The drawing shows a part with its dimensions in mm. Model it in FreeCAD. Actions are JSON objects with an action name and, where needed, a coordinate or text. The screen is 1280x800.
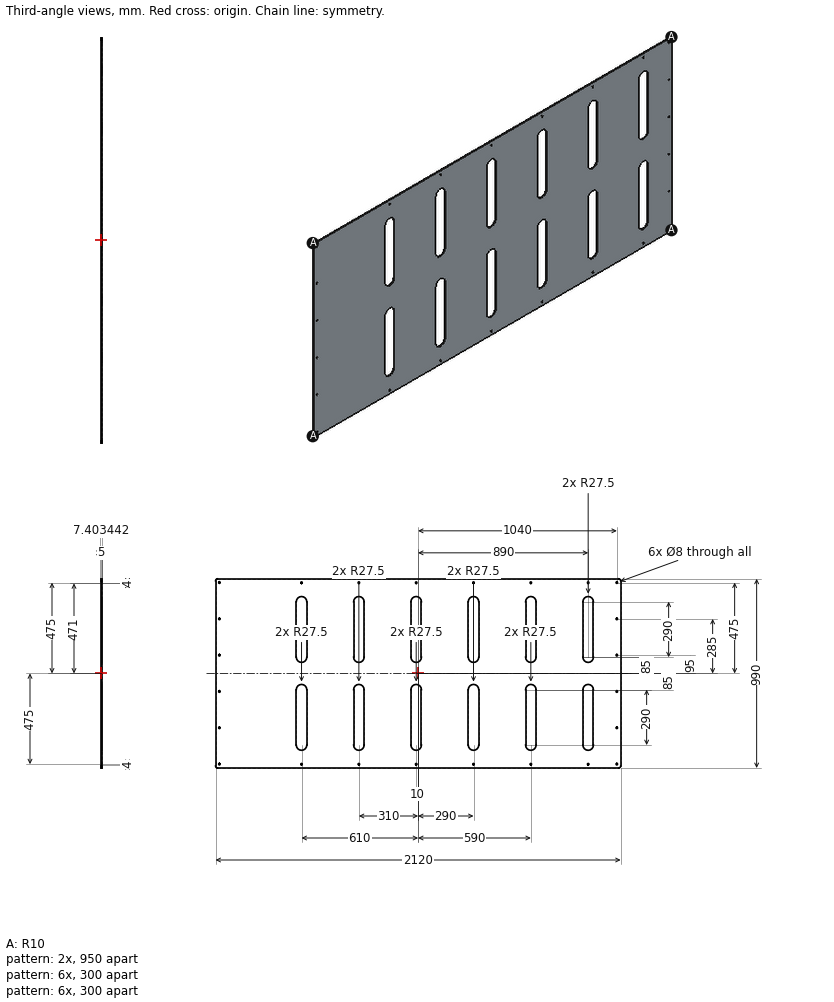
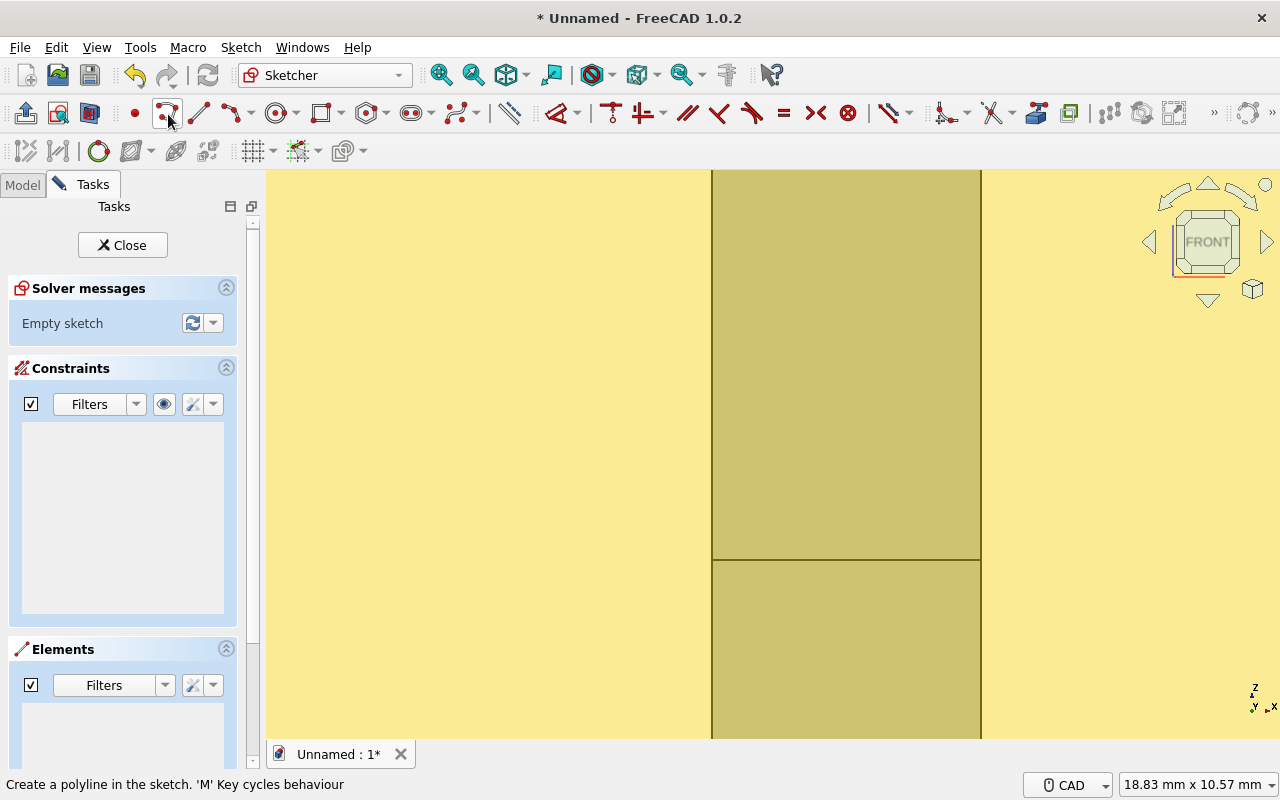
{"action": "left_click", "coordinate": [582, 345]}
{"action": "left_click", "coordinate": [981, 345]}
{"action": "left_click", "coordinate": [981, 560]}
{"action": "left_click", "coordinate": [712, 560]}
{"action": "left_click", "coordinate": [582, 346]}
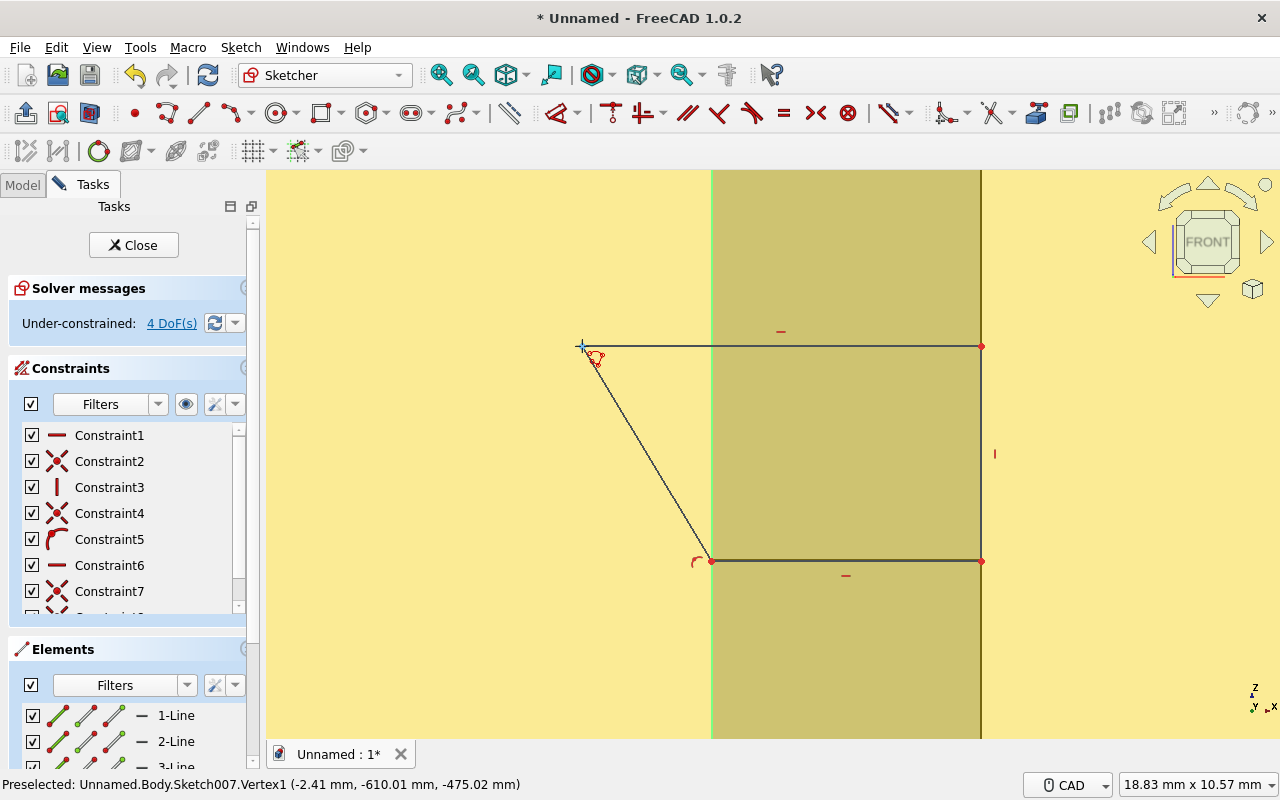
{"action": "left_click", "coordinate": [200, 114]}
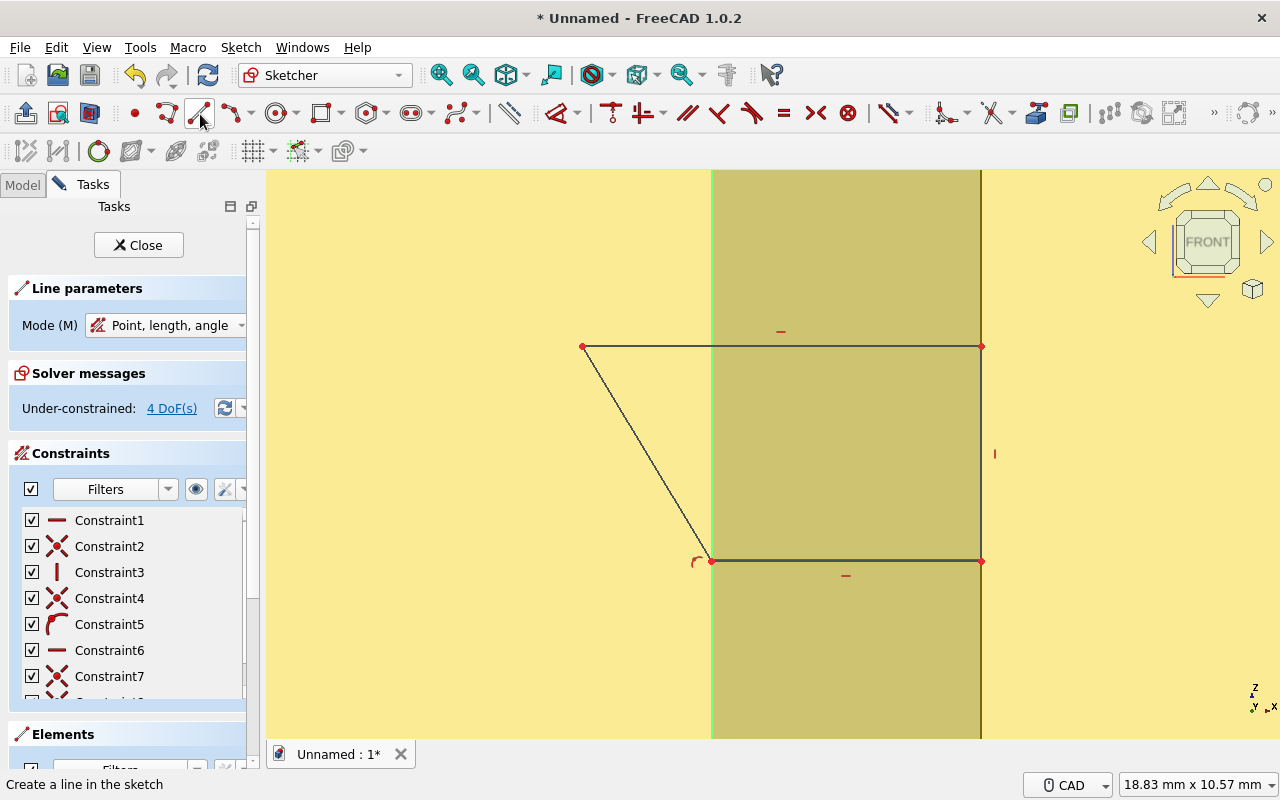
{"action": "left_click", "coordinate": [542, 345]}
{"action": "left_click", "coordinate": [423, 345]}
{"action": "key", "text": "Escape"}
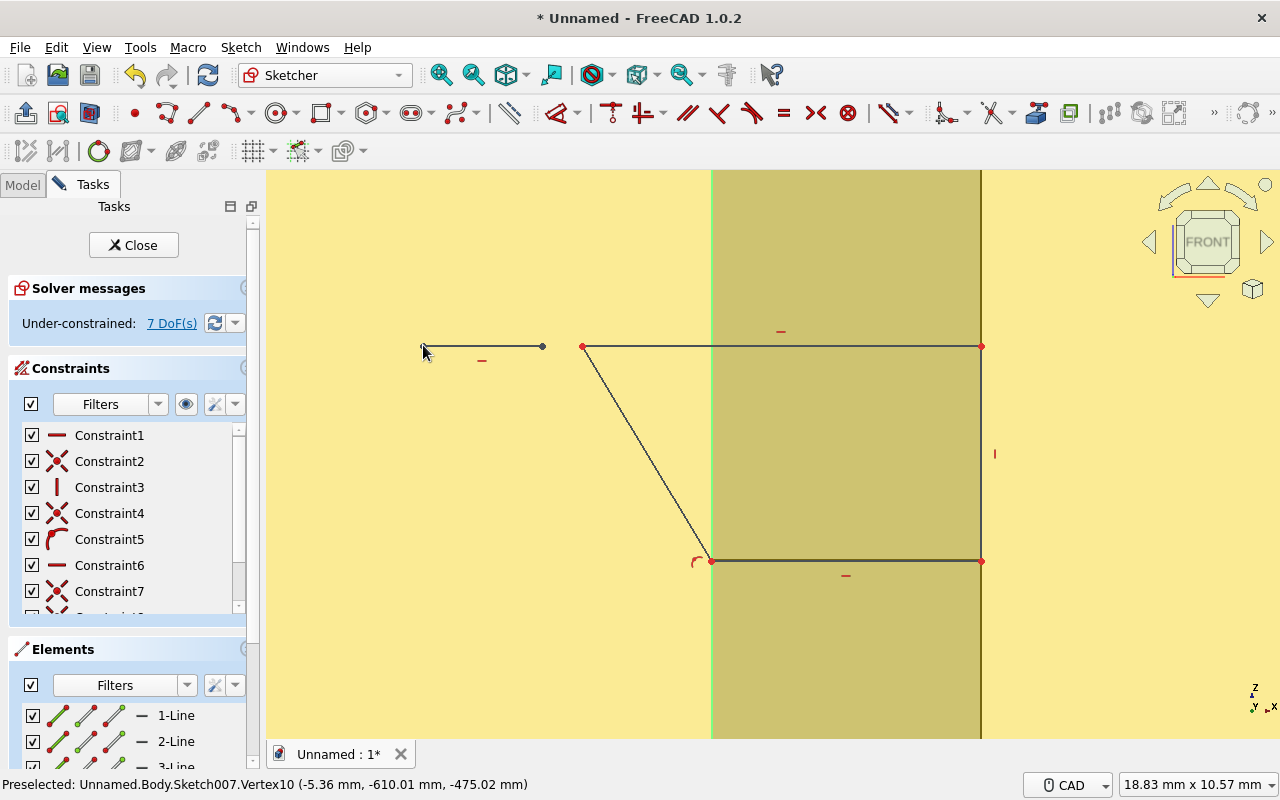
{"action": "left_click", "coordinate": [506, 346]}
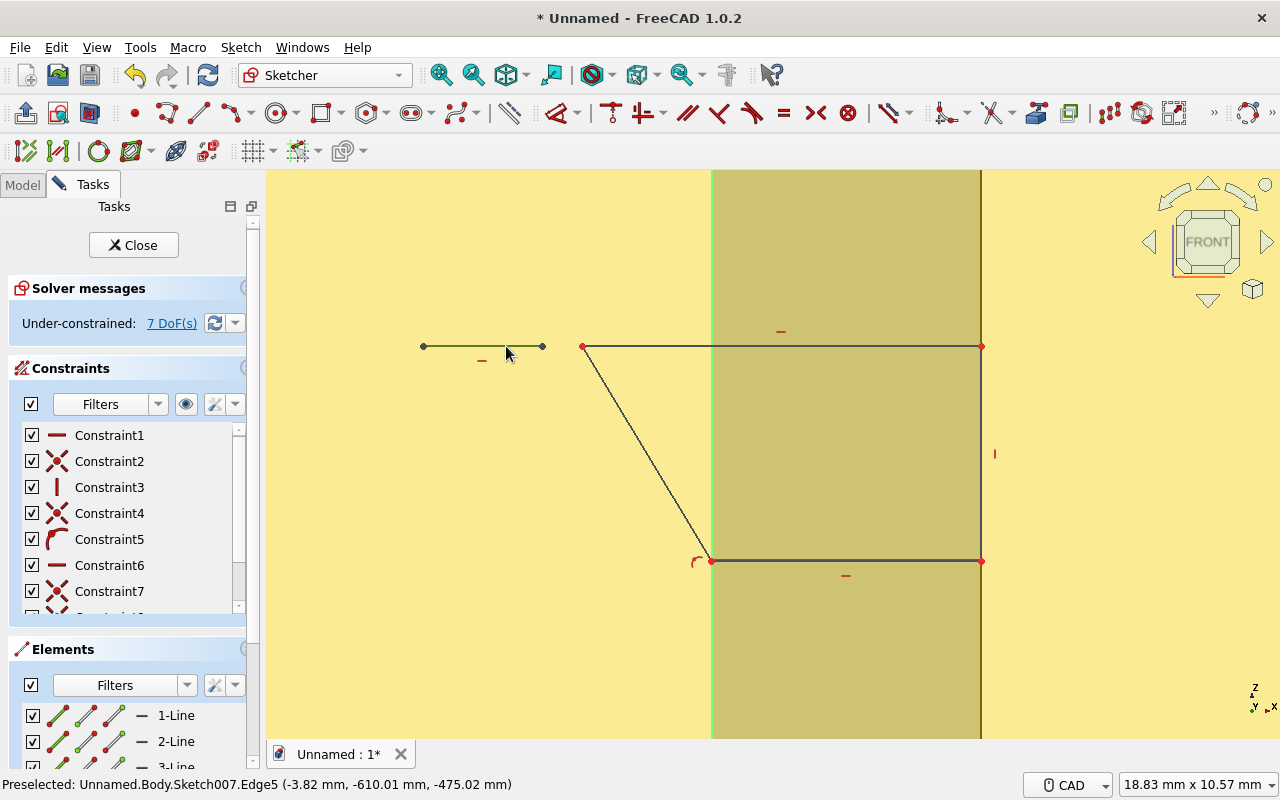
{"action": "left_click", "coordinate": [510, 114]}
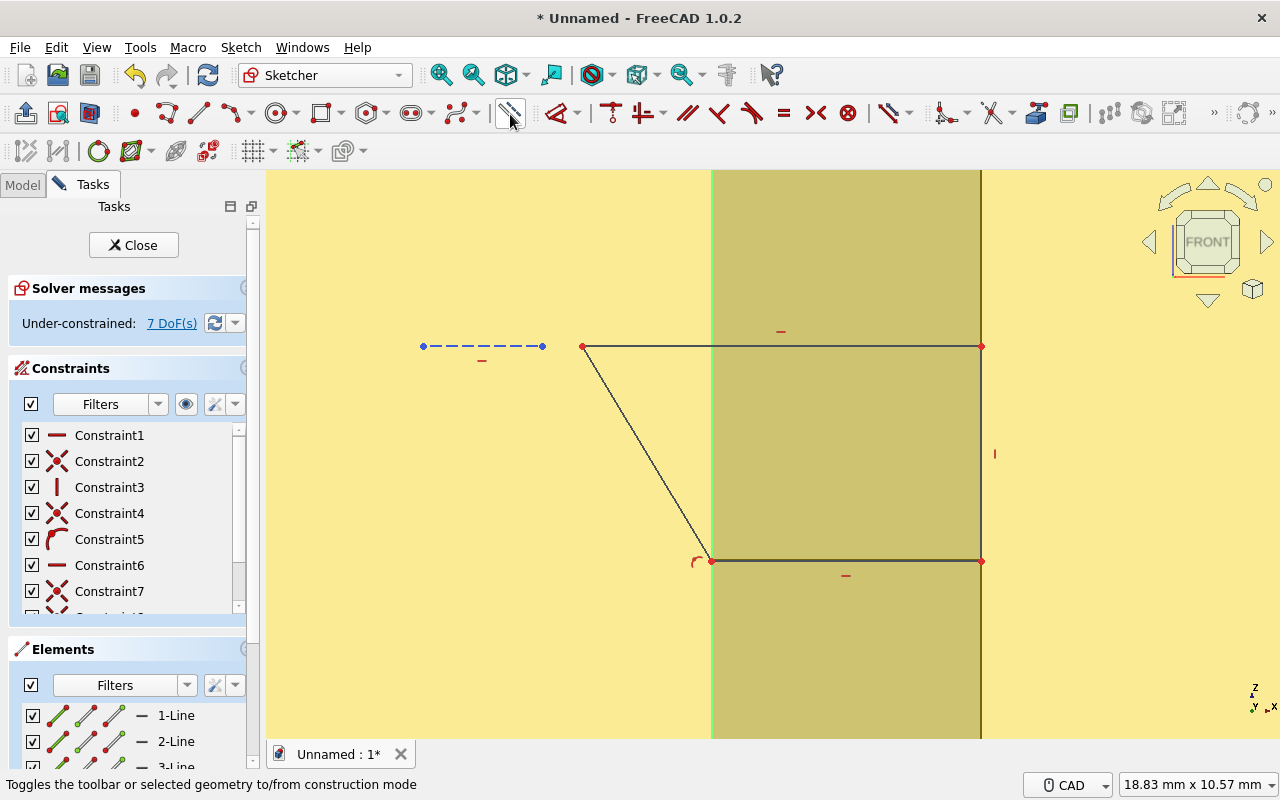
{"action": "left_click", "coordinate": [556, 114]}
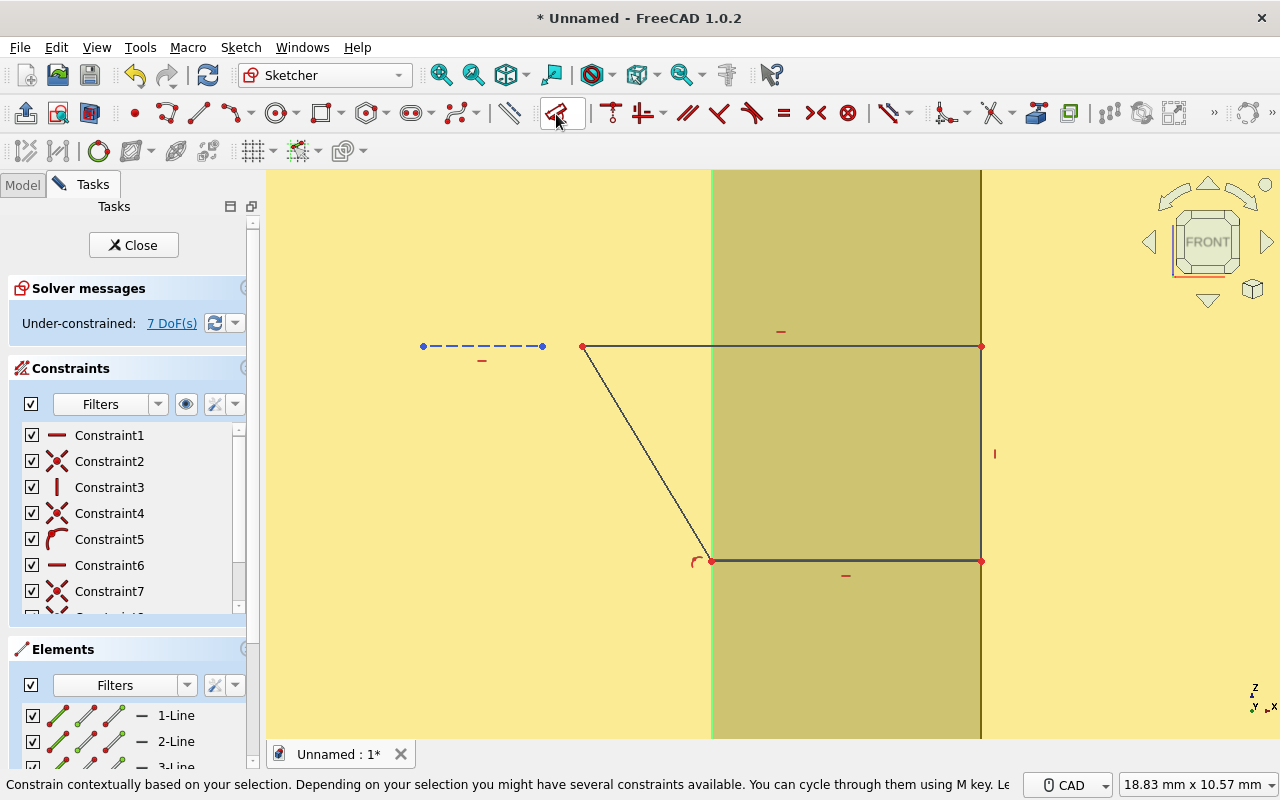
{"action": "left_click", "coordinate": [981, 411]}
{"action": "left_click", "coordinate": [1015, 454]}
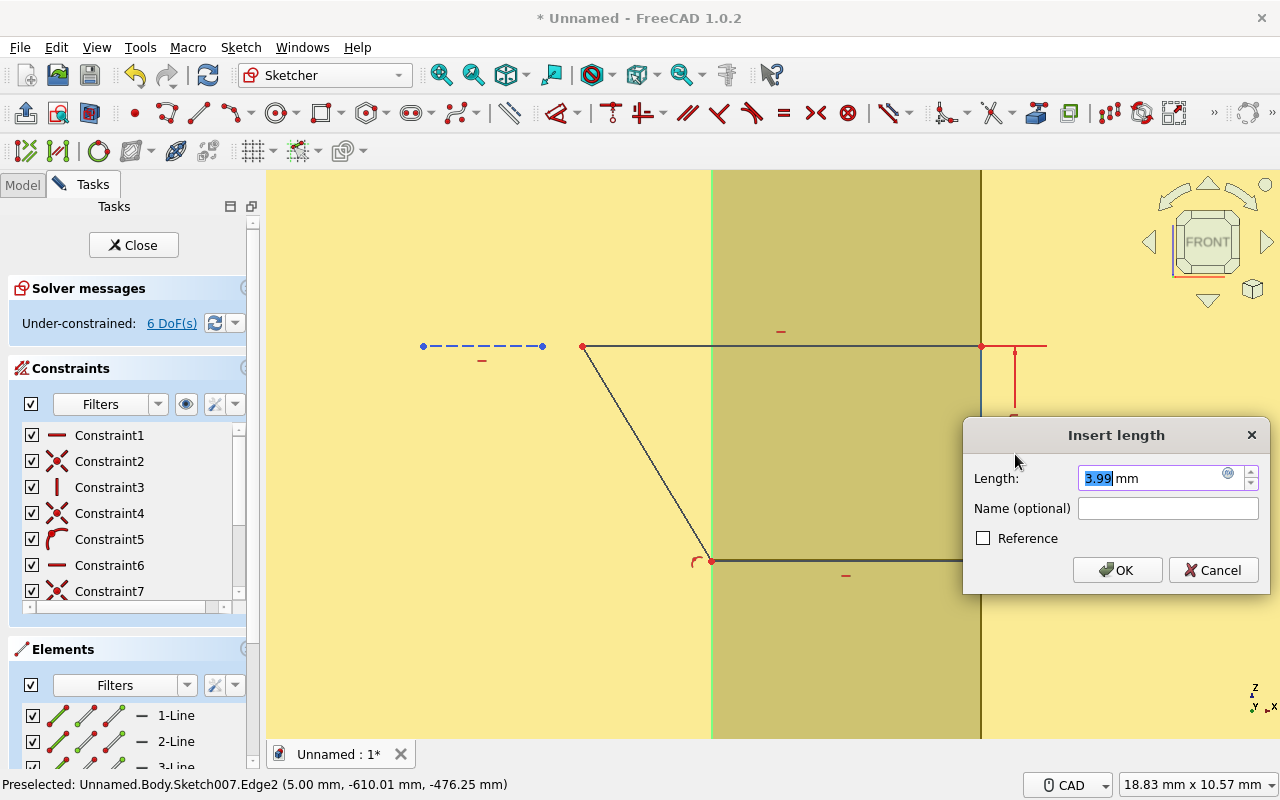
{"action": "type", "text": "4"}
{"action": "key", "text": "Return"}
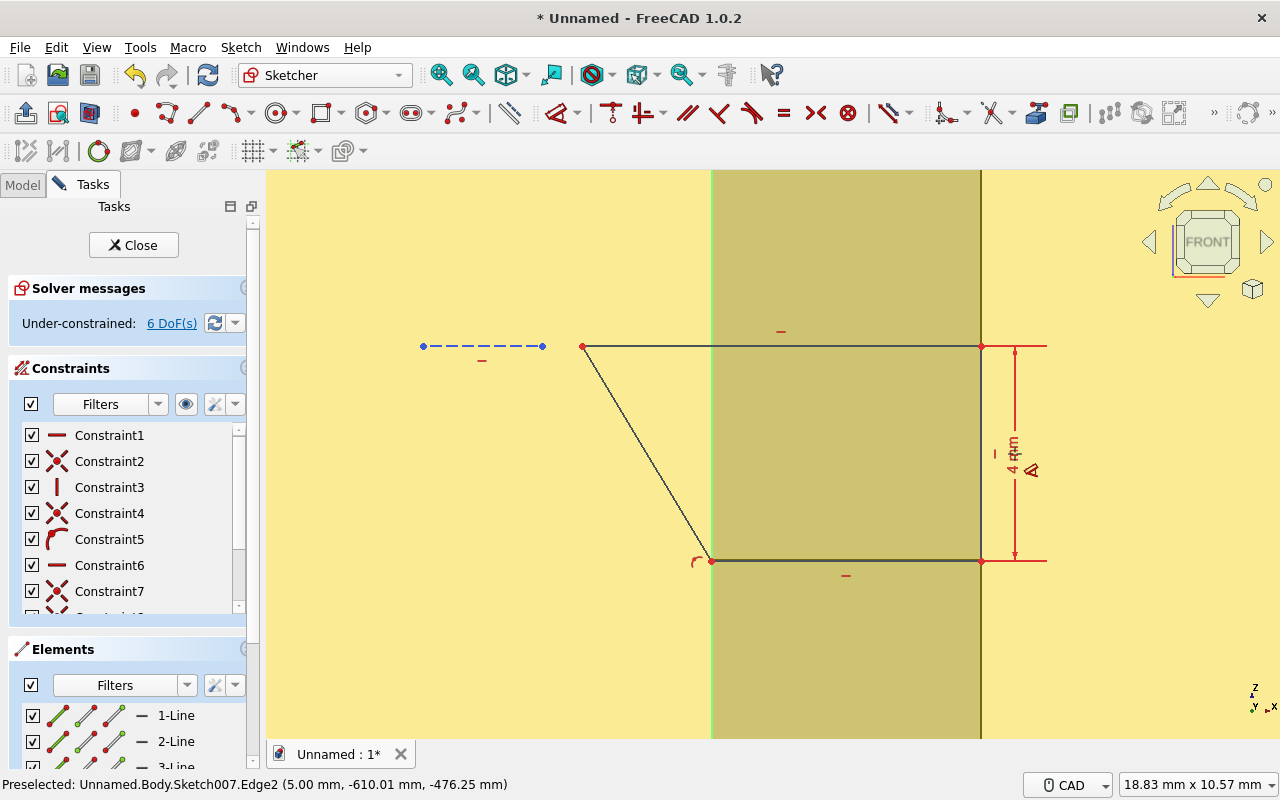
{"action": "left_click", "coordinate": [900, 561]}
{"action": "left_click", "coordinate": [846, 595]}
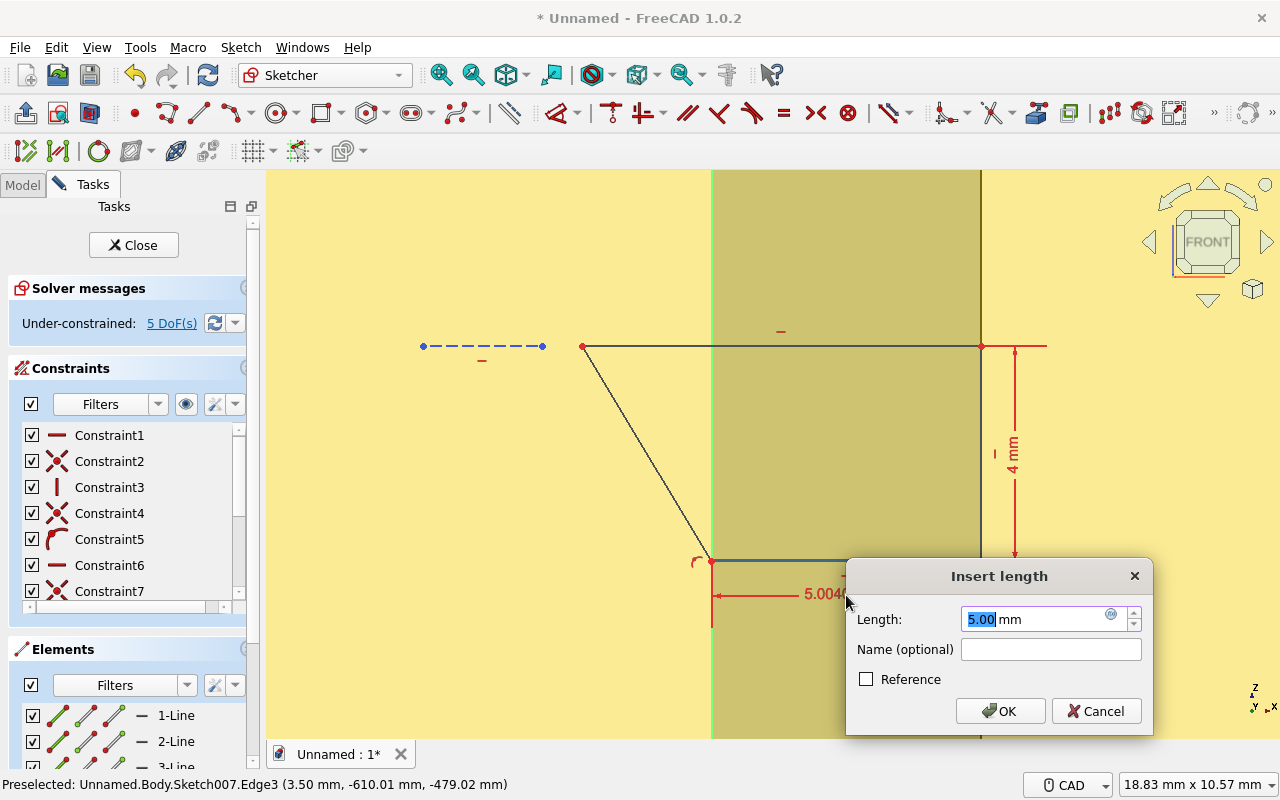
{"action": "type", "text": "5"}
{"action": "key", "text": "Return"}